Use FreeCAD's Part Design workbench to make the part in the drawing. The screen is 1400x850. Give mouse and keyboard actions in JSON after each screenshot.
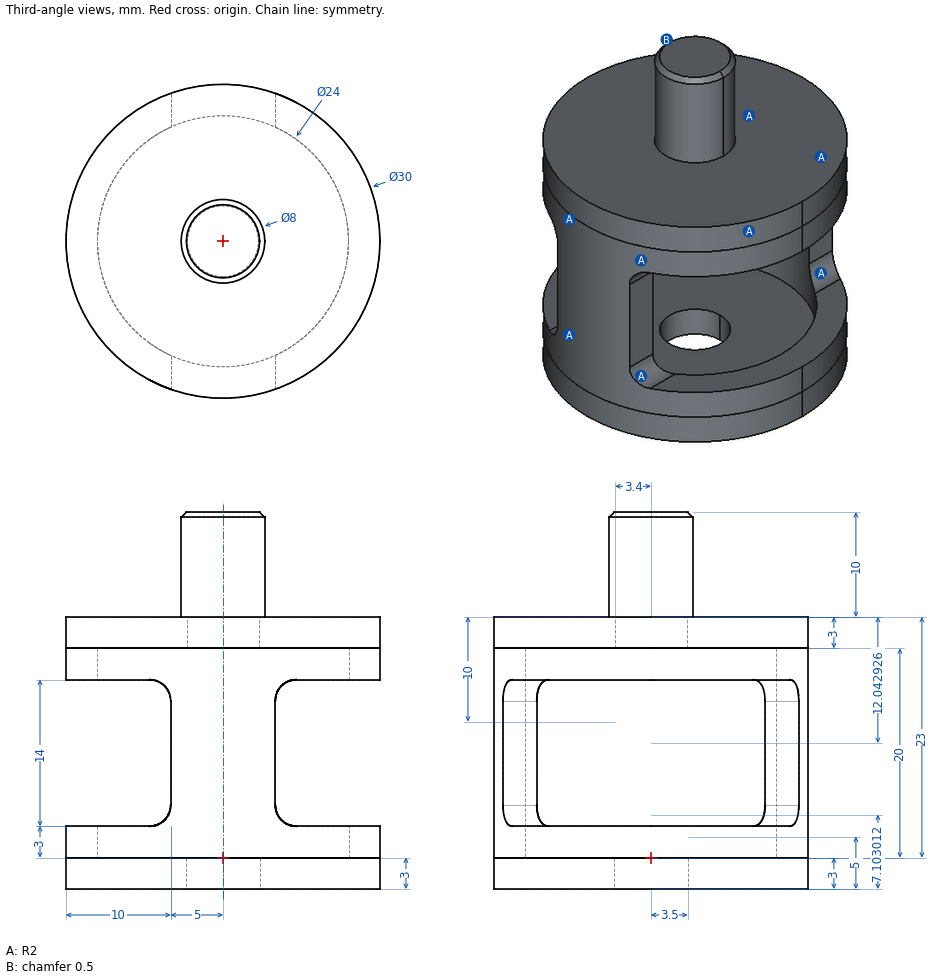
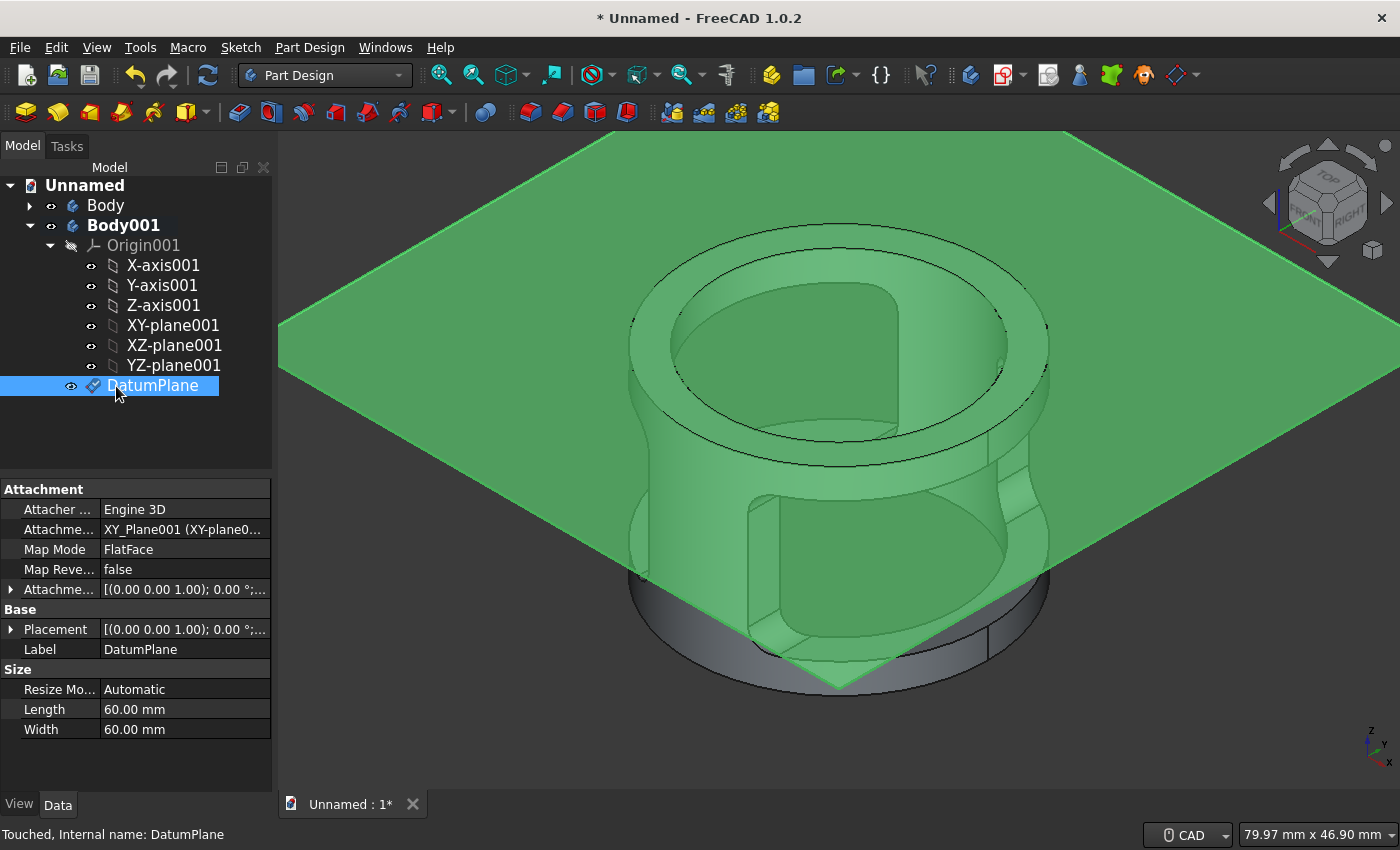
{"action": "left_click", "coordinate": [1004, 76]}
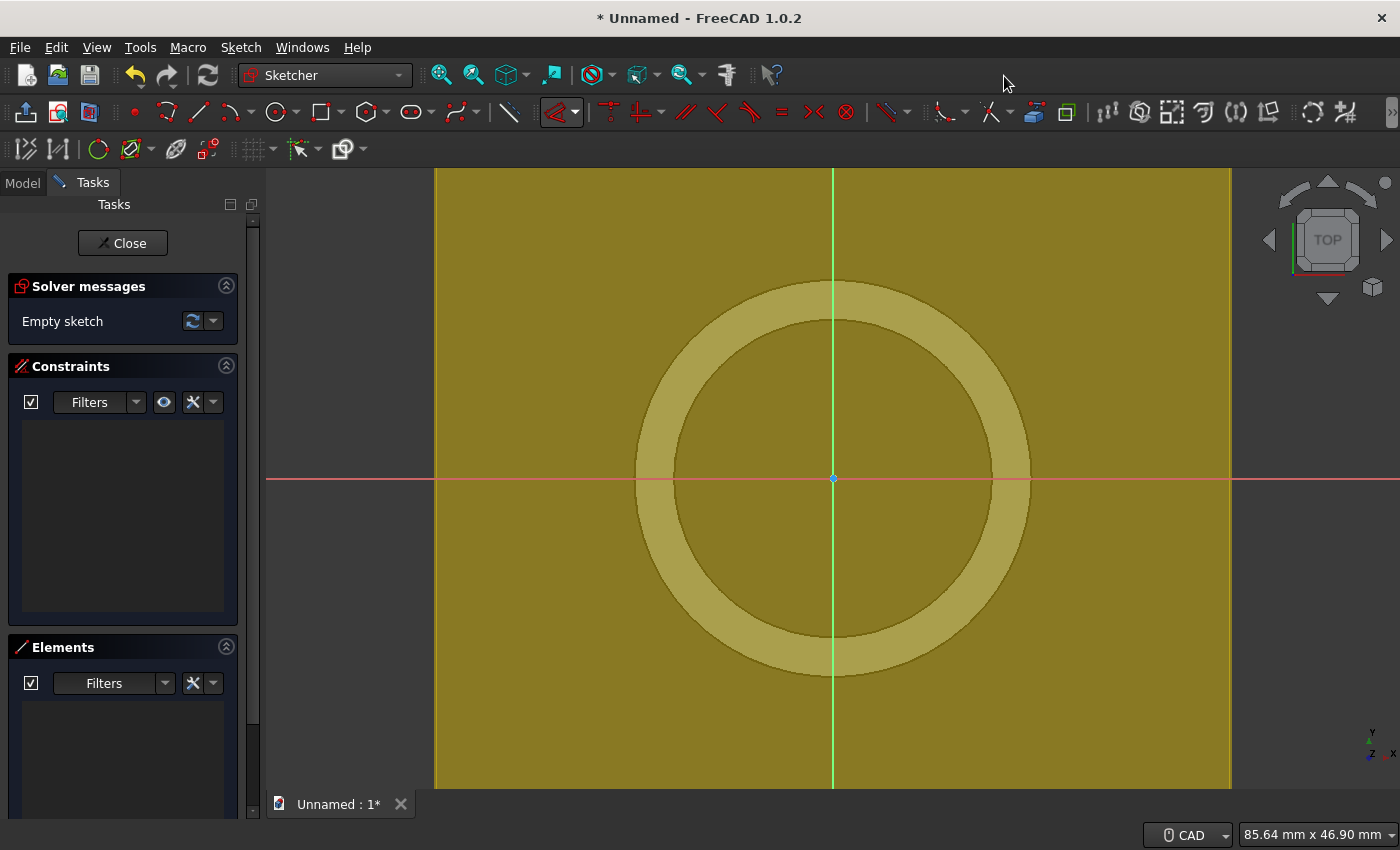
{"action": "key", "text": "g c"}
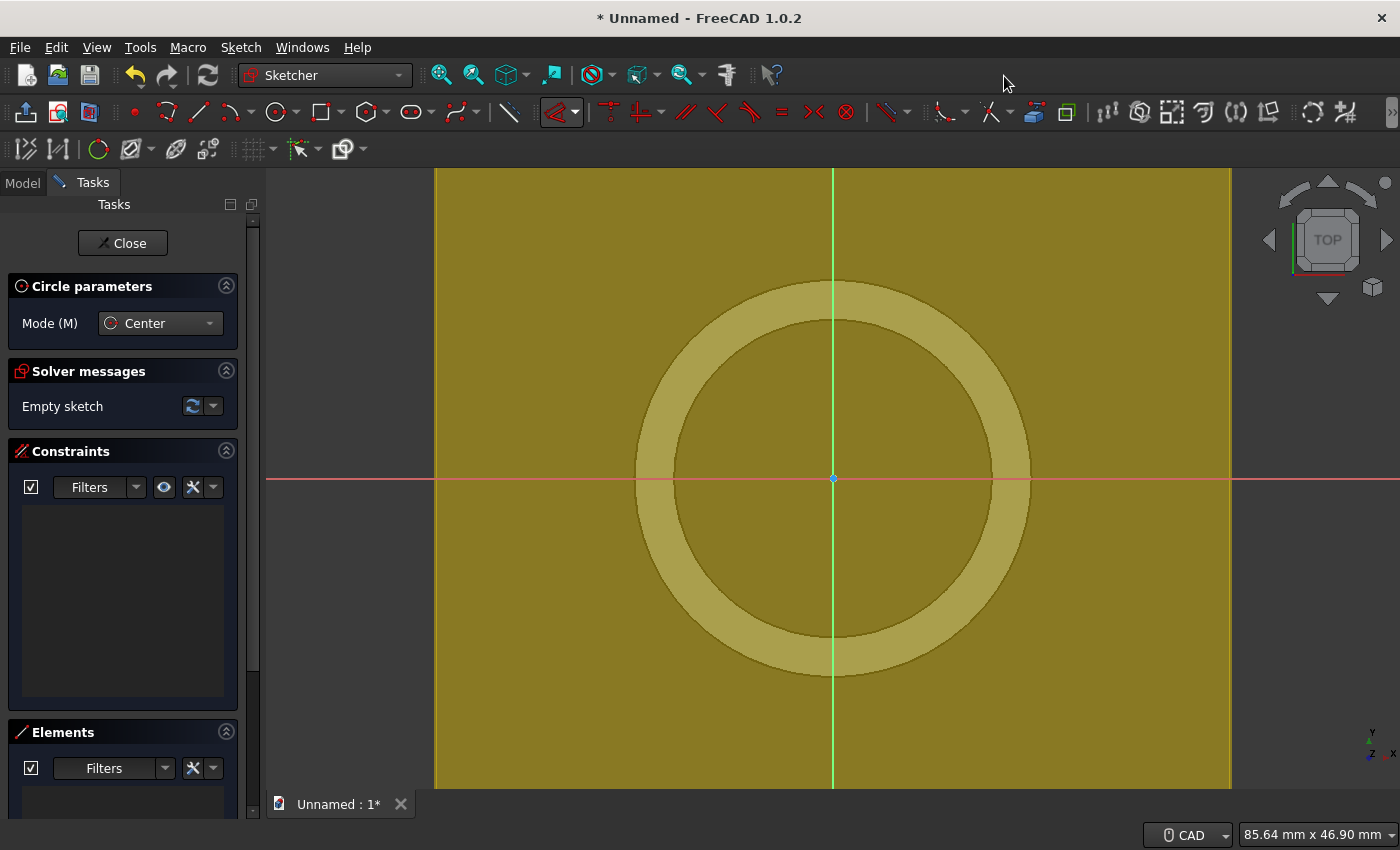
{"action": "left_click", "coordinate": [833, 478]}
{"action": "left_click", "coordinate": [973, 338]}
{"action": "key", "text": "Escape"}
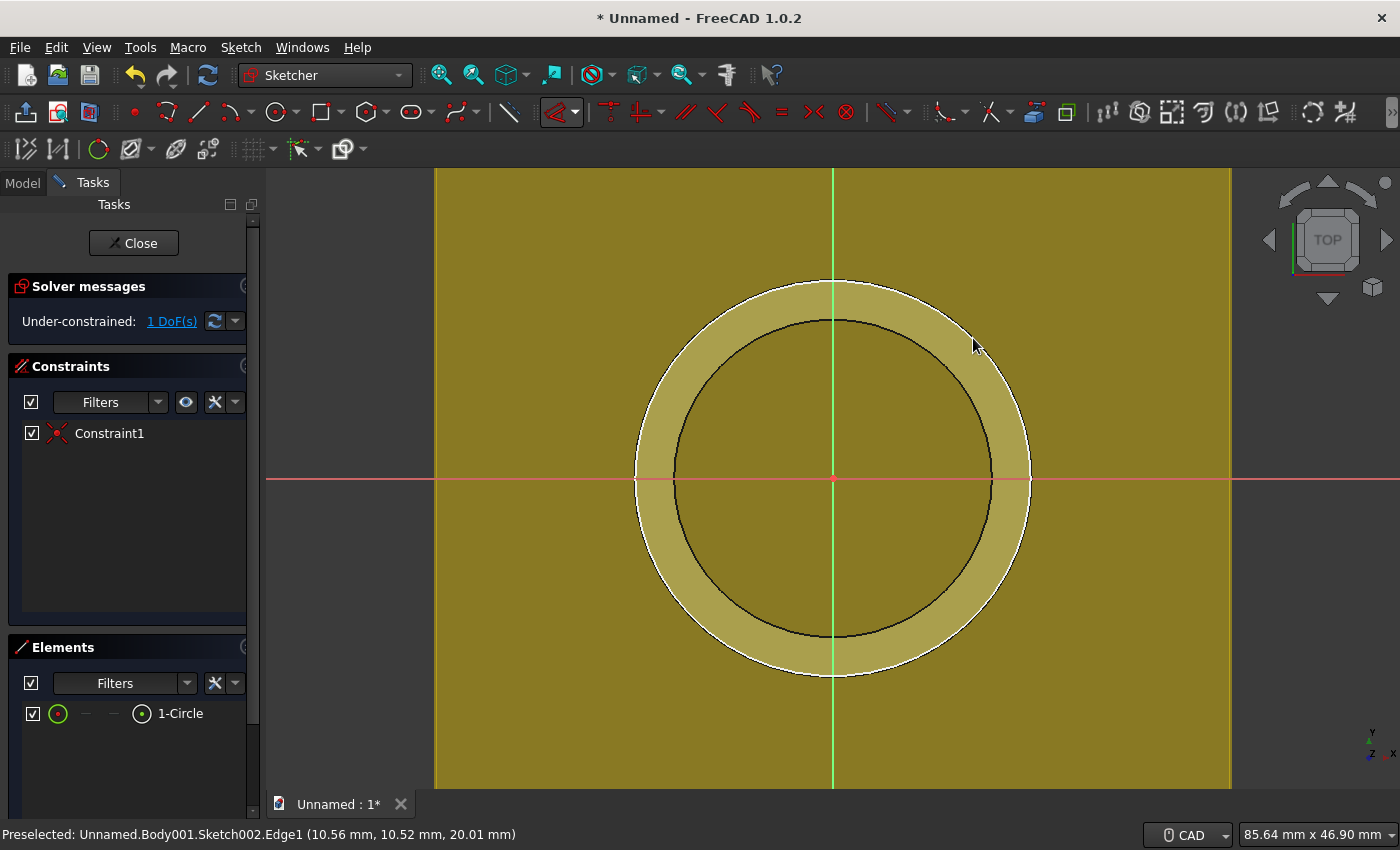
{"action": "left_click", "coordinate": [972, 338]}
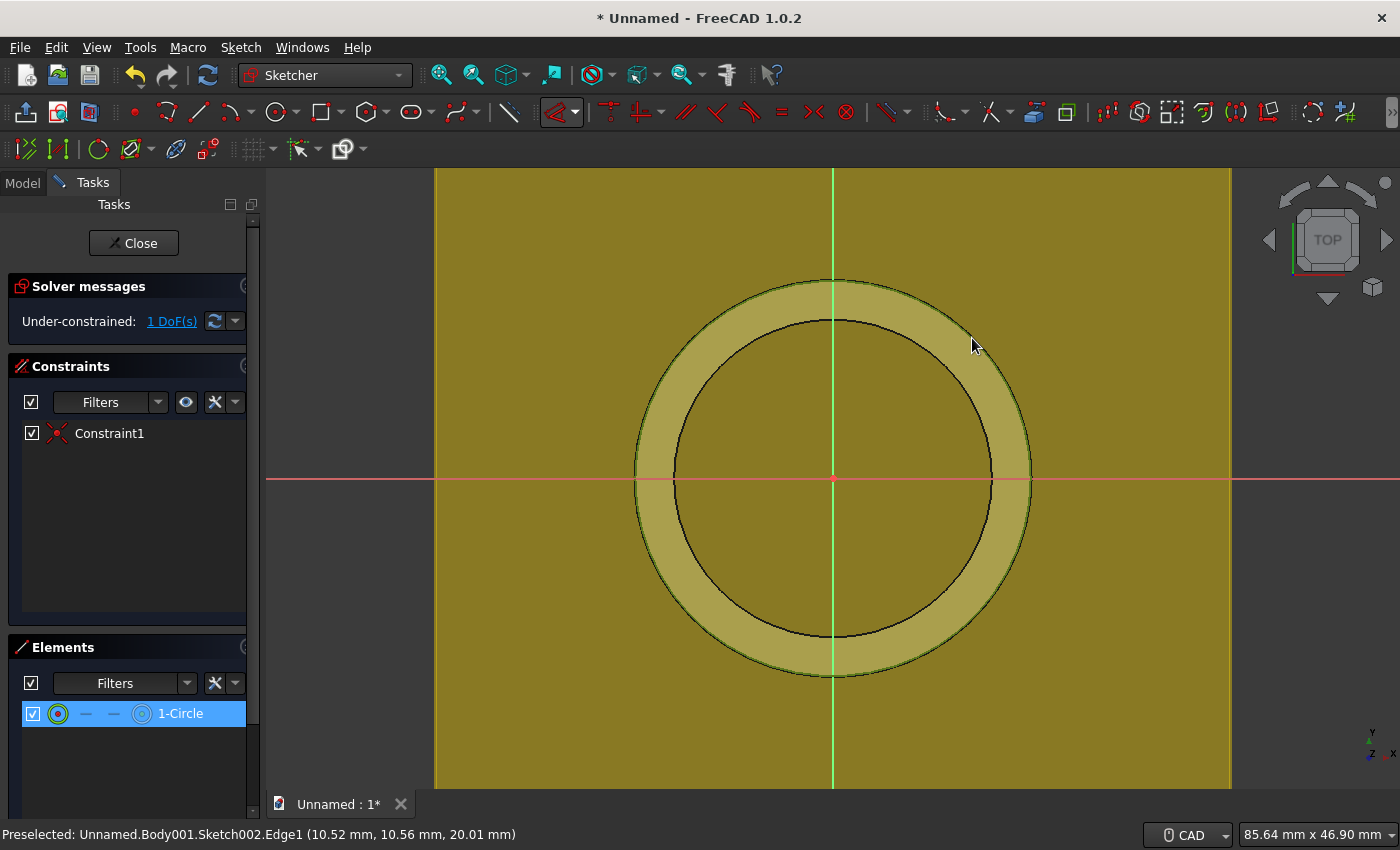
{"action": "key", "text": "k o"}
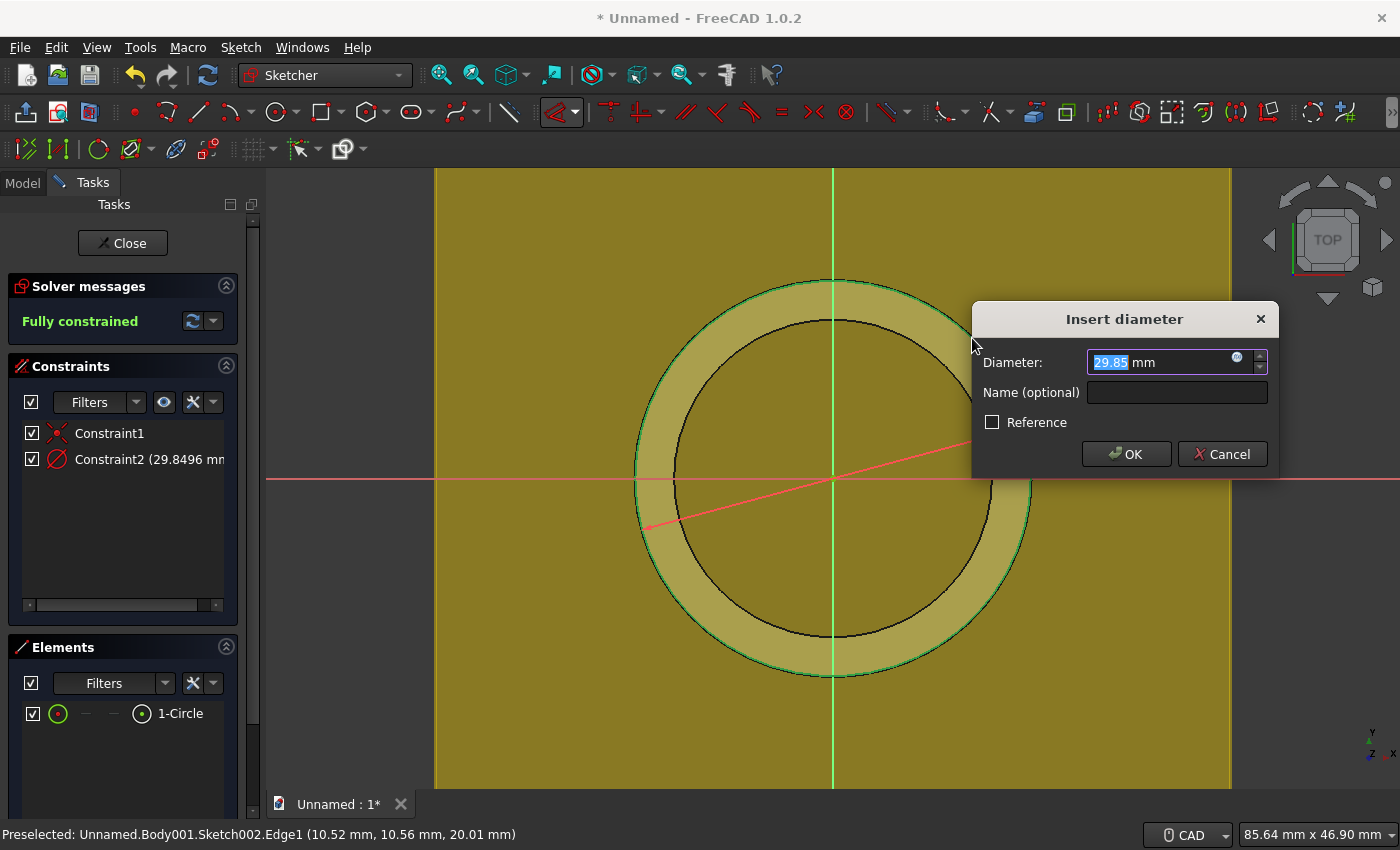
{"action": "type", "text": "30"}
{"action": "key", "text": "Return"}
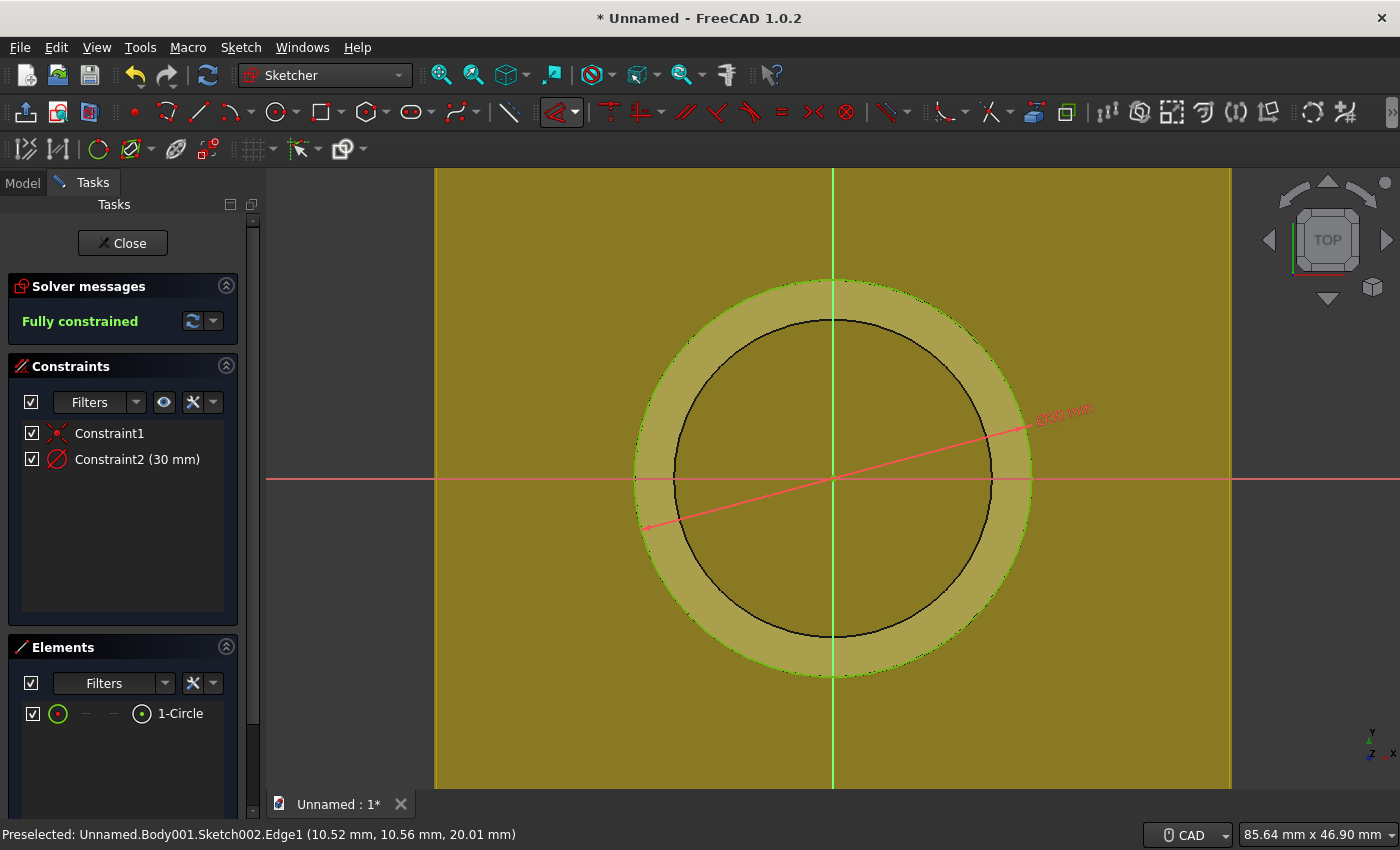
{"action": "left_click", "coordinate": [123, 243]}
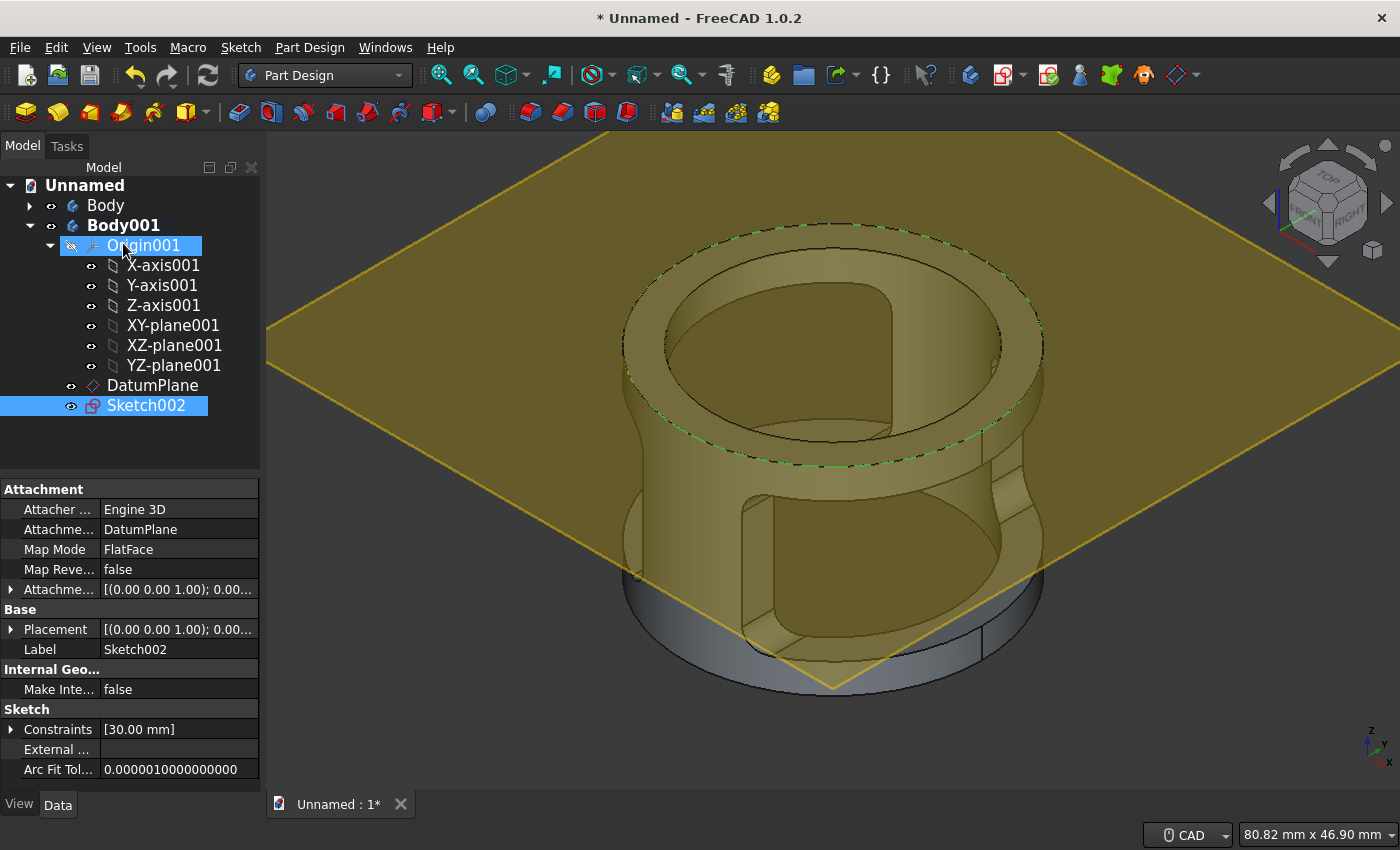
{"action": "left_click", "coordinate": [26, 112]}